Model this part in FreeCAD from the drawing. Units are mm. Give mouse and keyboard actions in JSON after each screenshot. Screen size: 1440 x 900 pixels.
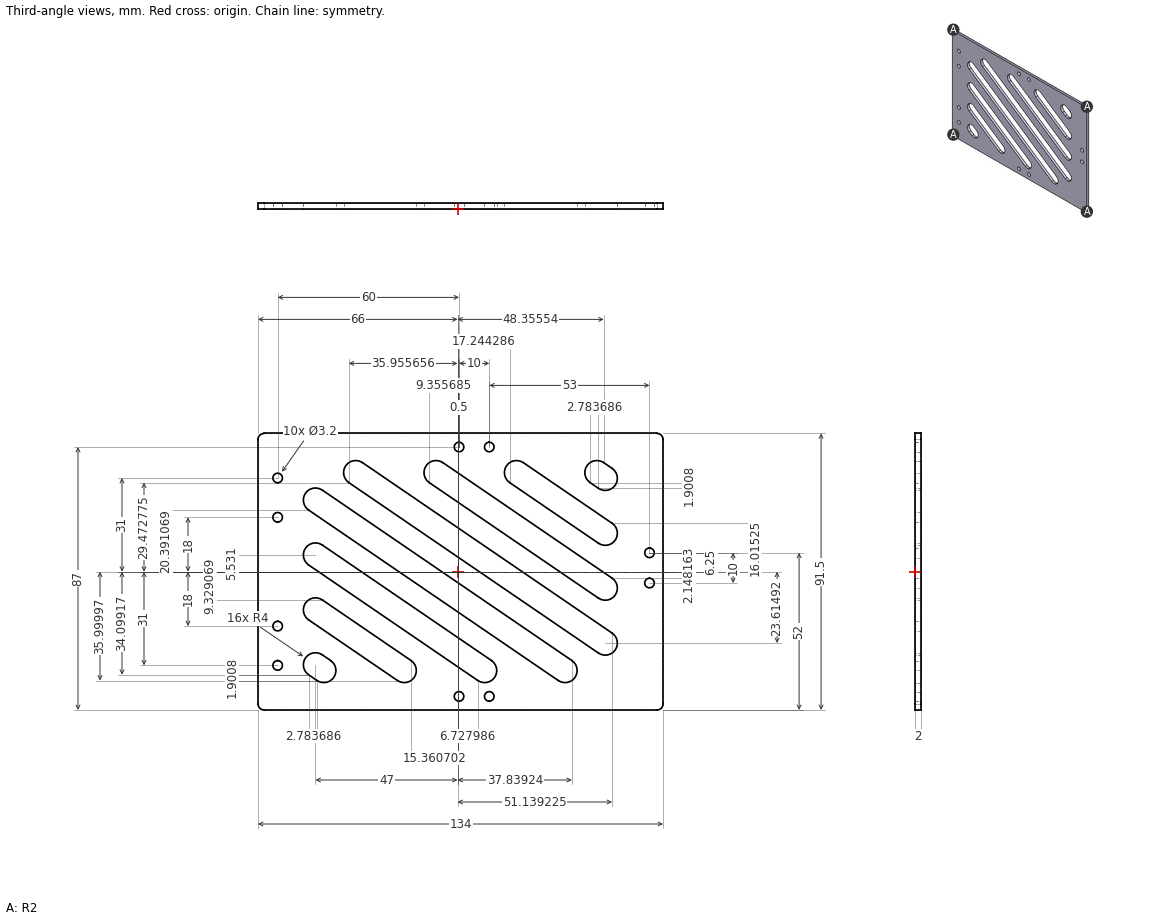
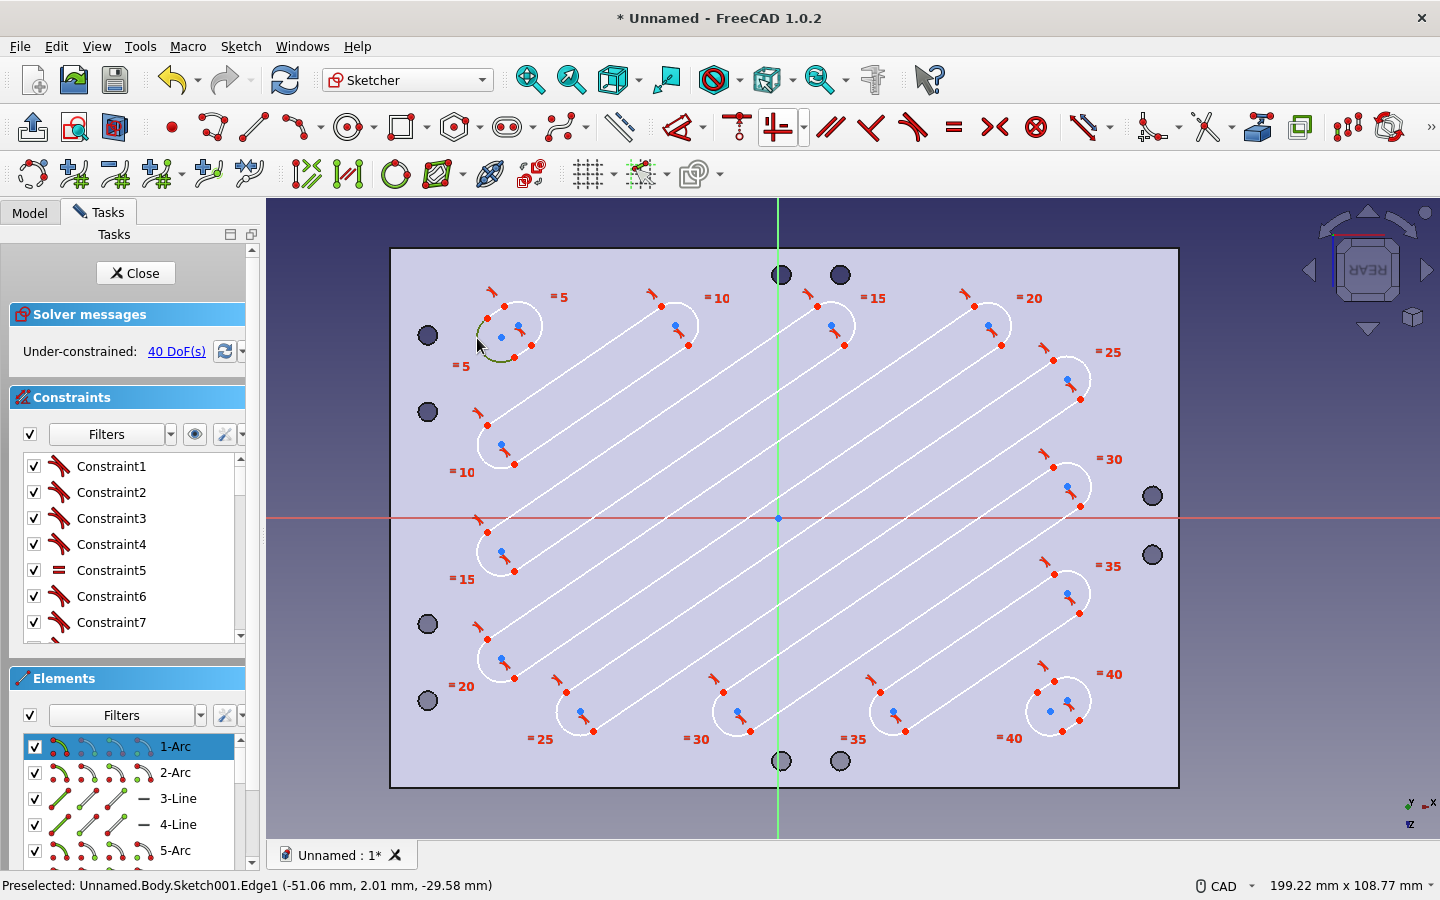
{"action": "left_click", "coordinate": [478, 444]}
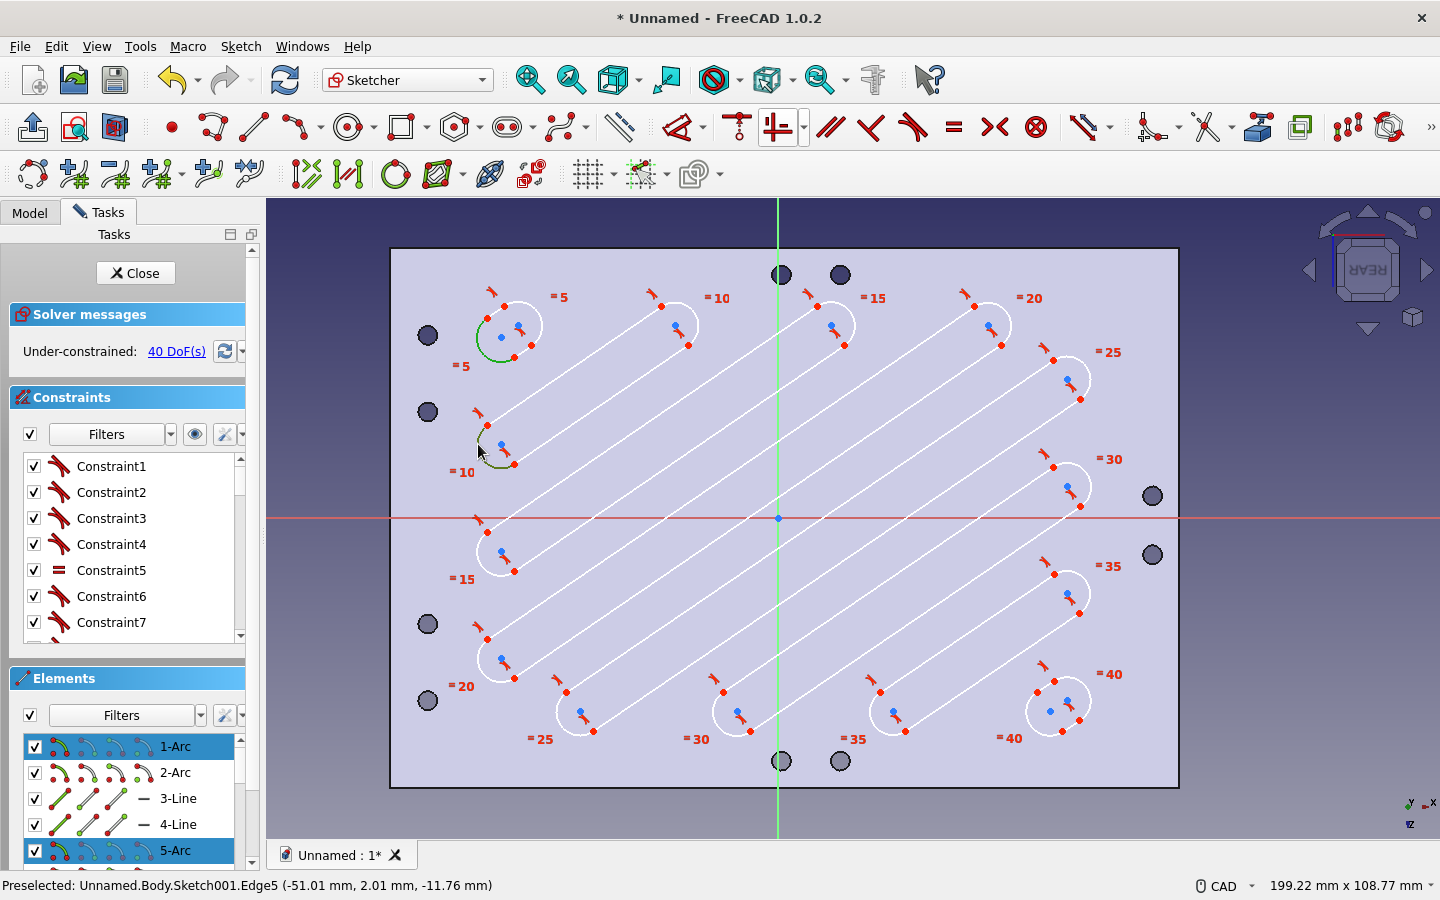
{"action": "left_click", "coordinate": [477, 551]}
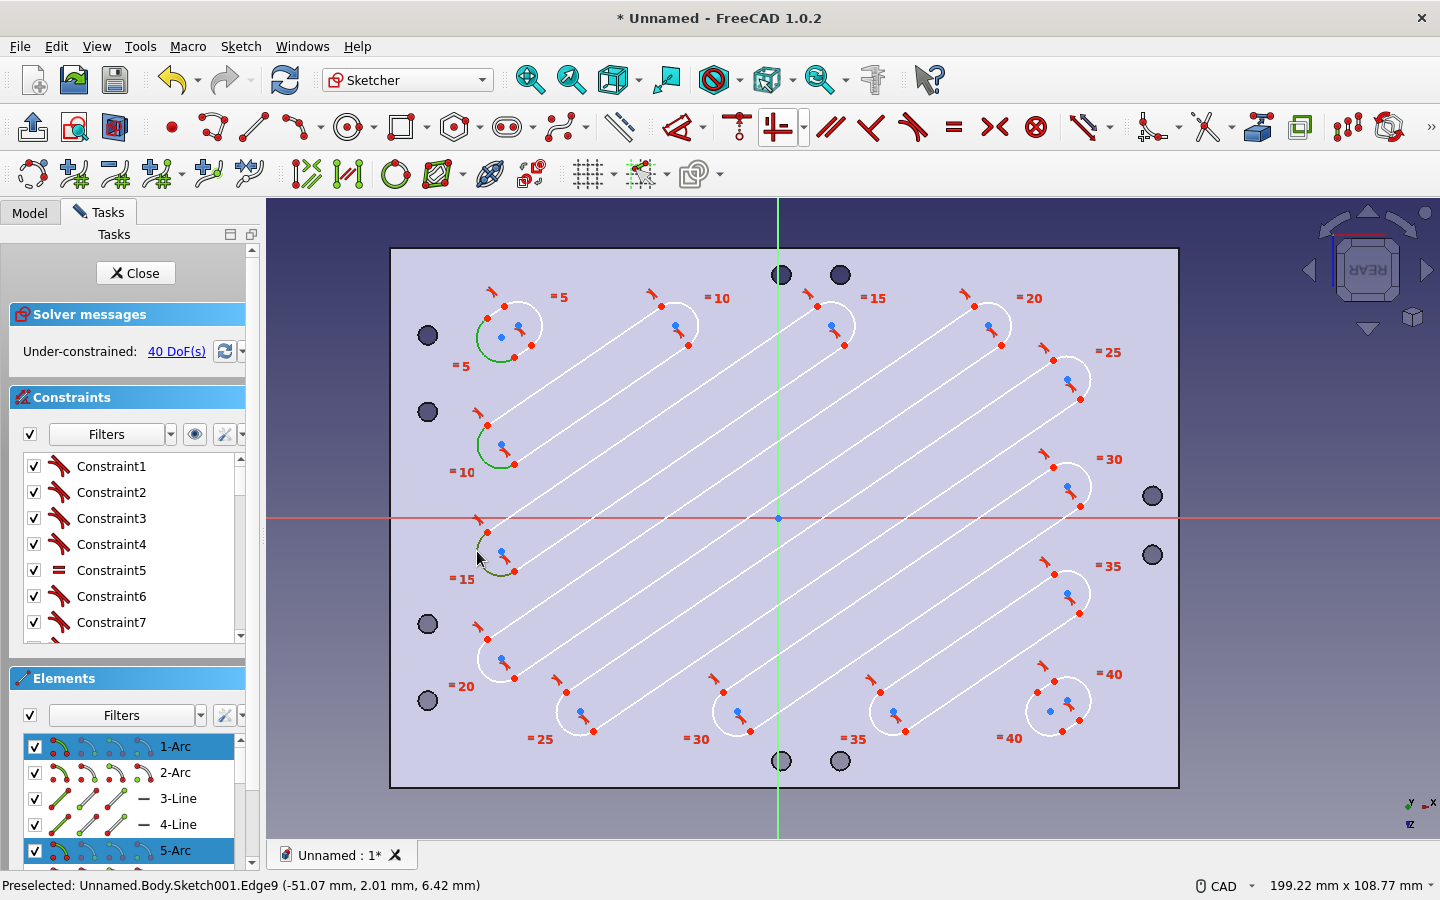
{"action": "left_click", "coordinate": [478, 658]}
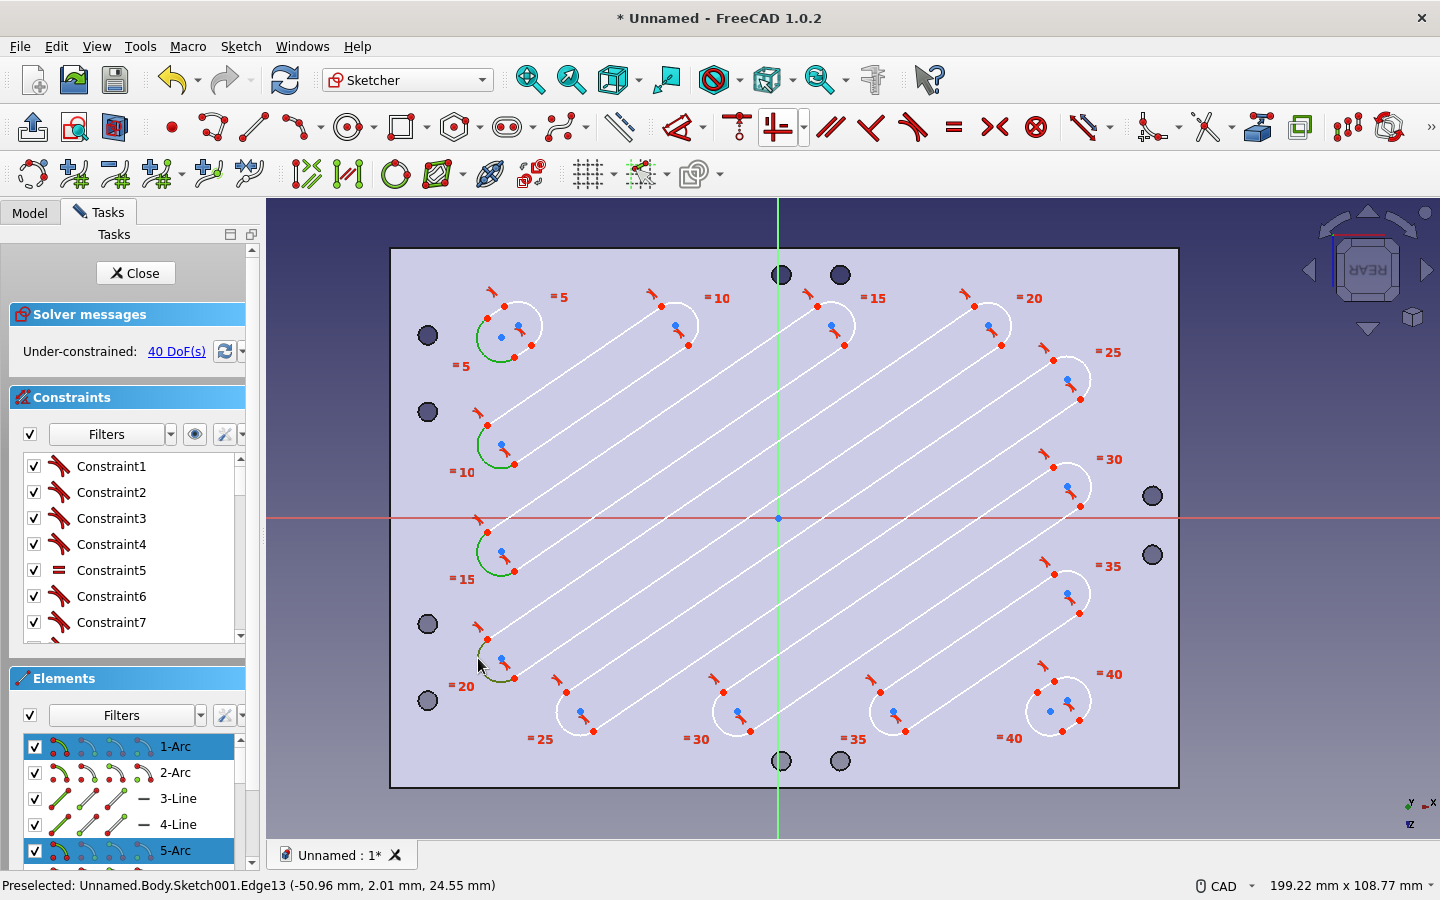
{"action": "left_click", "coordinate": [557, 711]}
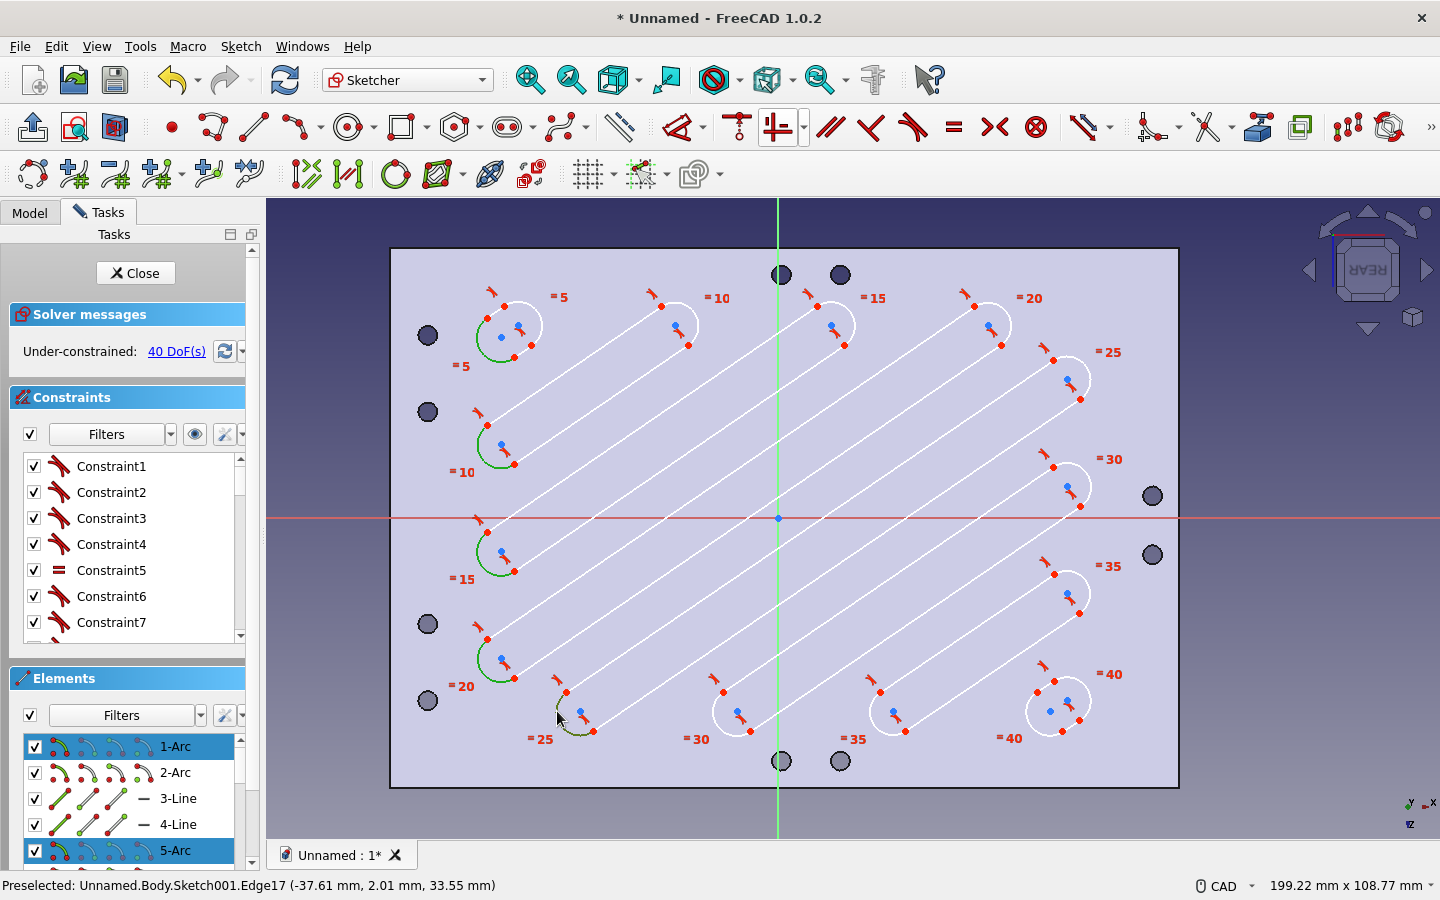
{"action": "left_click", "coordinate": [713, 711]}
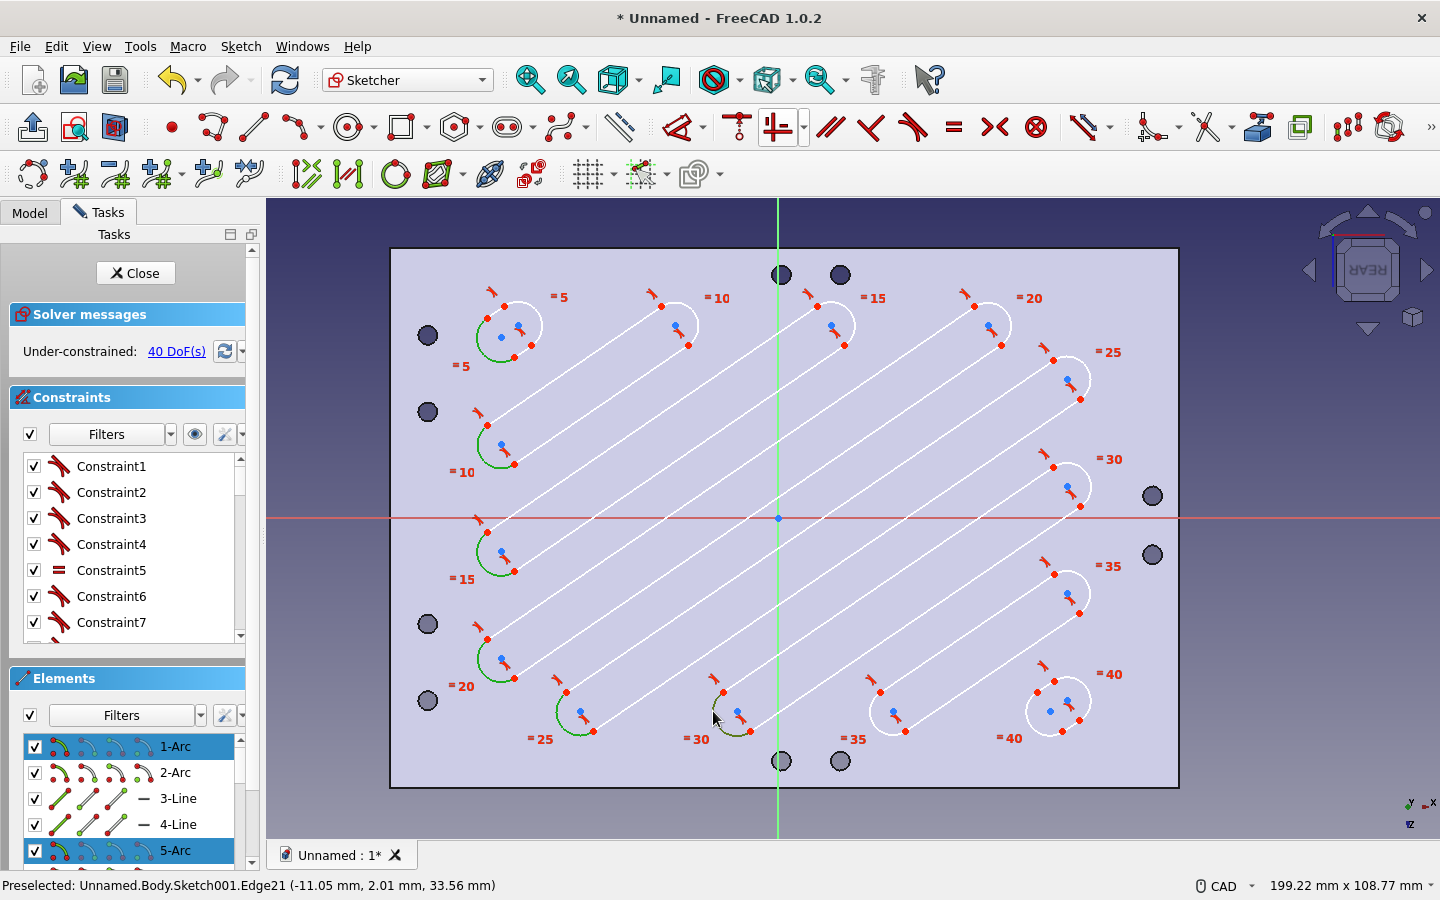
{"action": "left_click", "coordinate": [870, 711]}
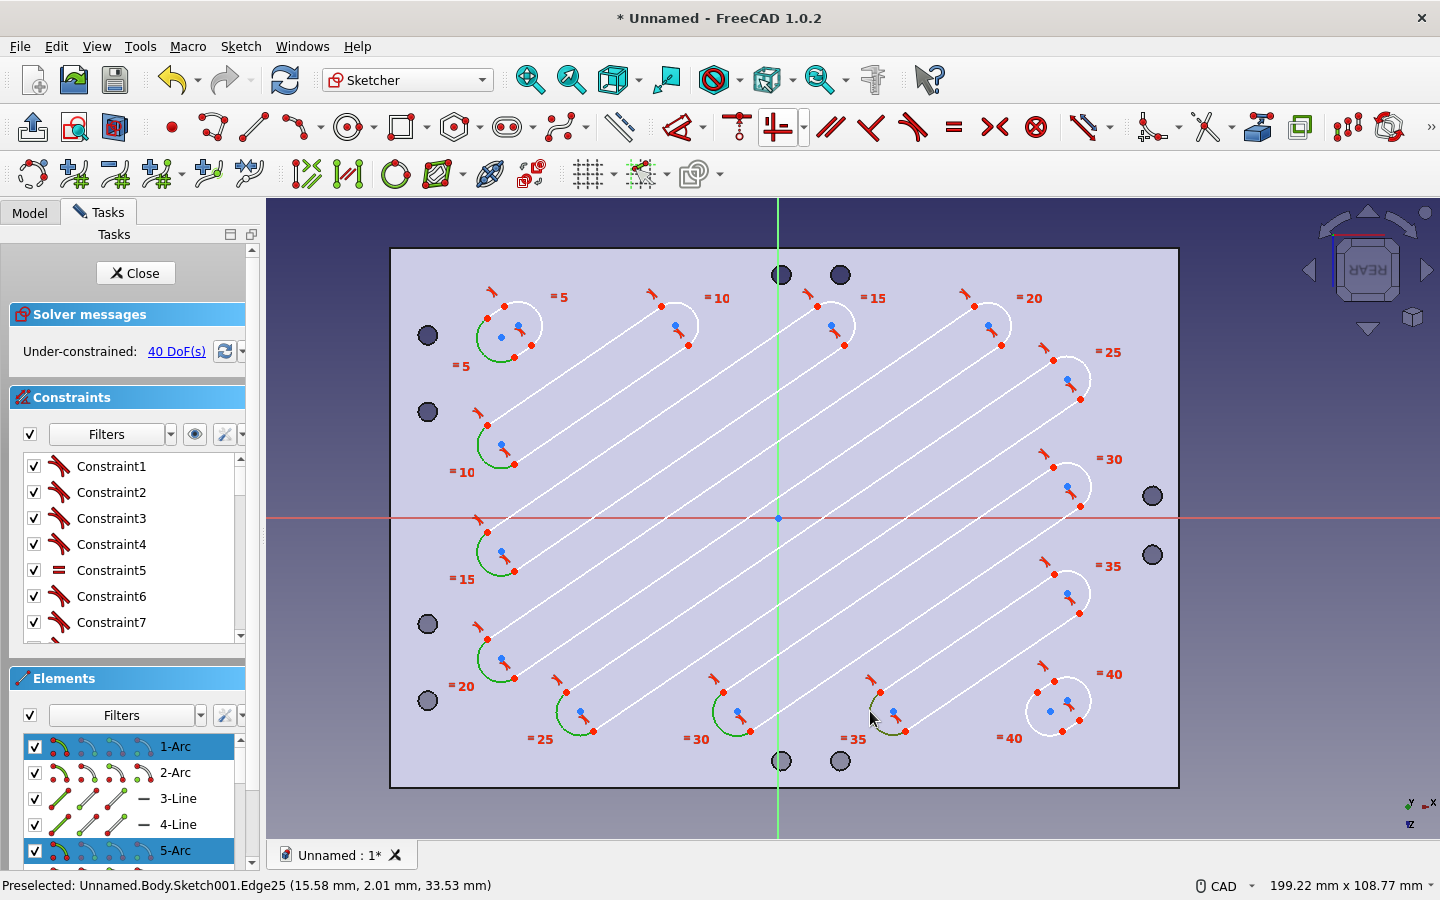
{"action": "left_click", "coordinate": [1026, 711]}